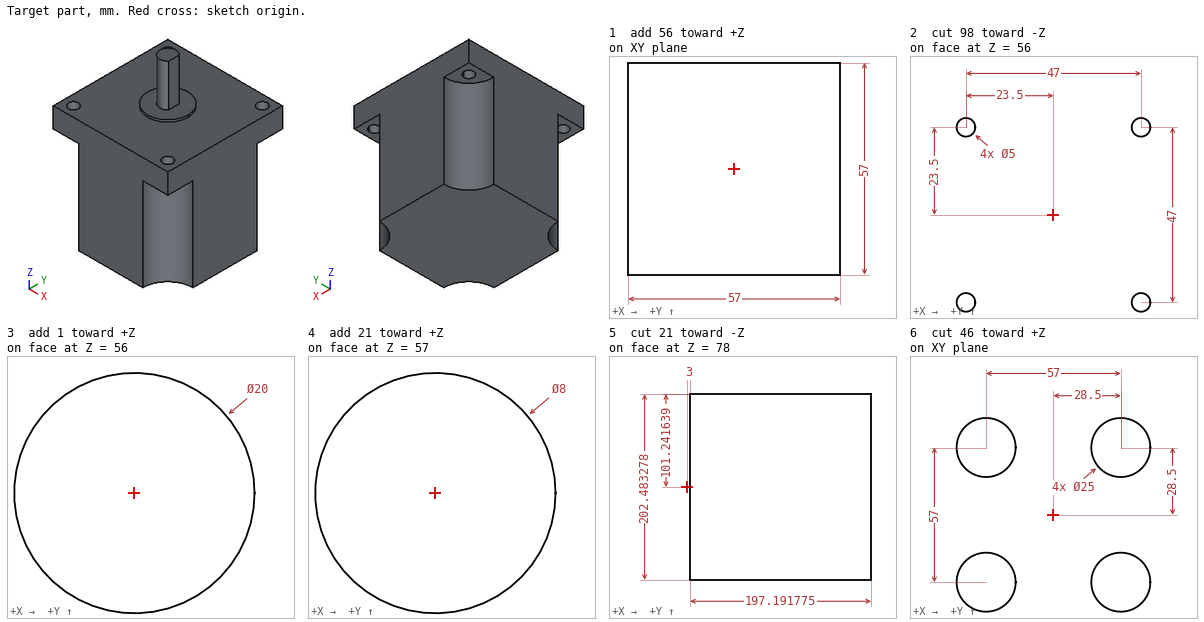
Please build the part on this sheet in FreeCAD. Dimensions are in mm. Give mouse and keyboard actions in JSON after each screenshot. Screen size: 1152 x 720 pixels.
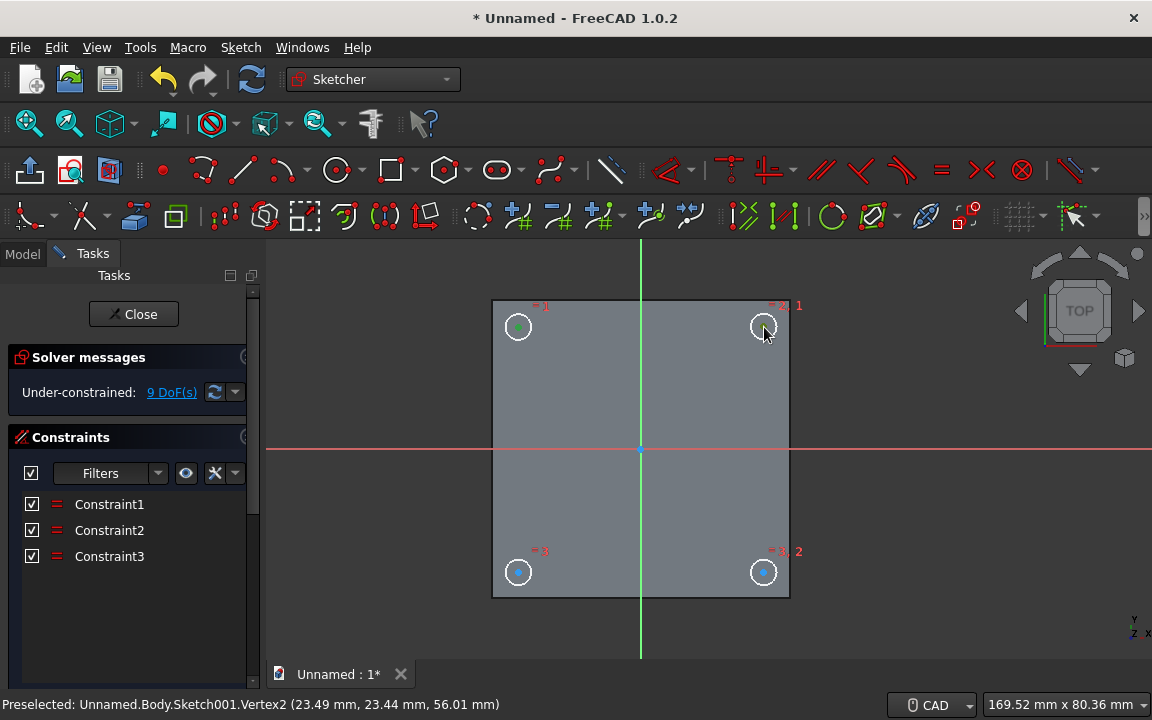
{"action": "key", "text": "h"}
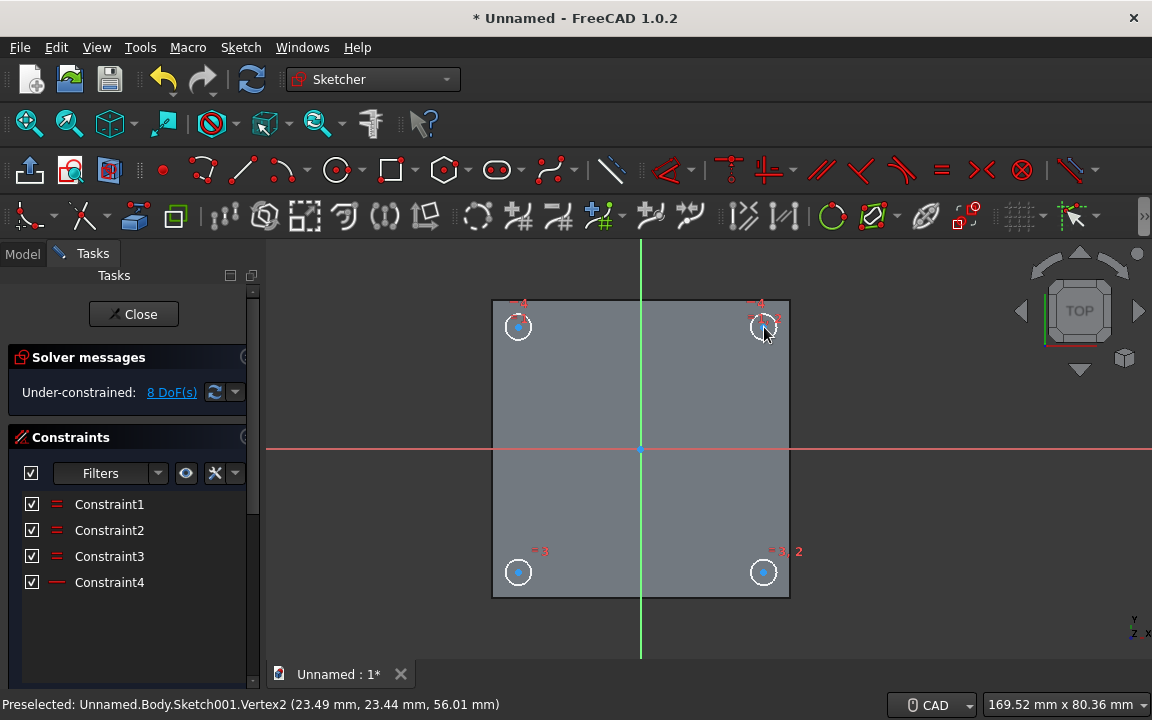
{"action": "left_click", "coordinate": [764, 327]}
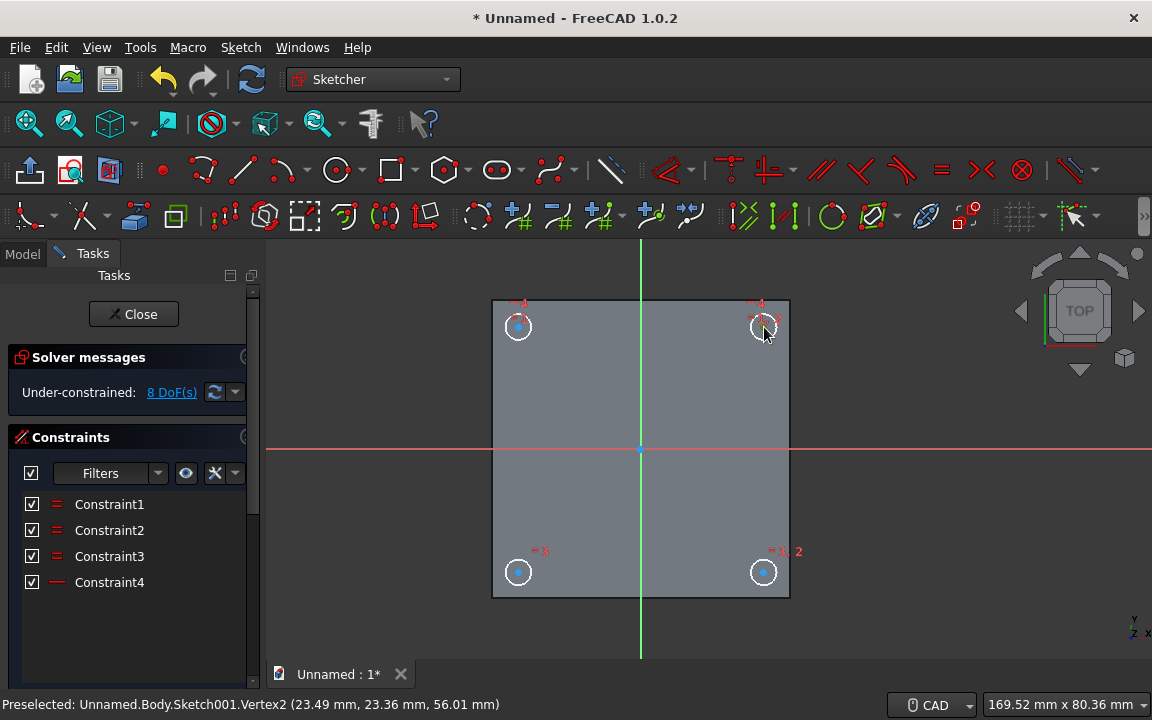
{"action": "left_click", "coordinate": [764, 572]}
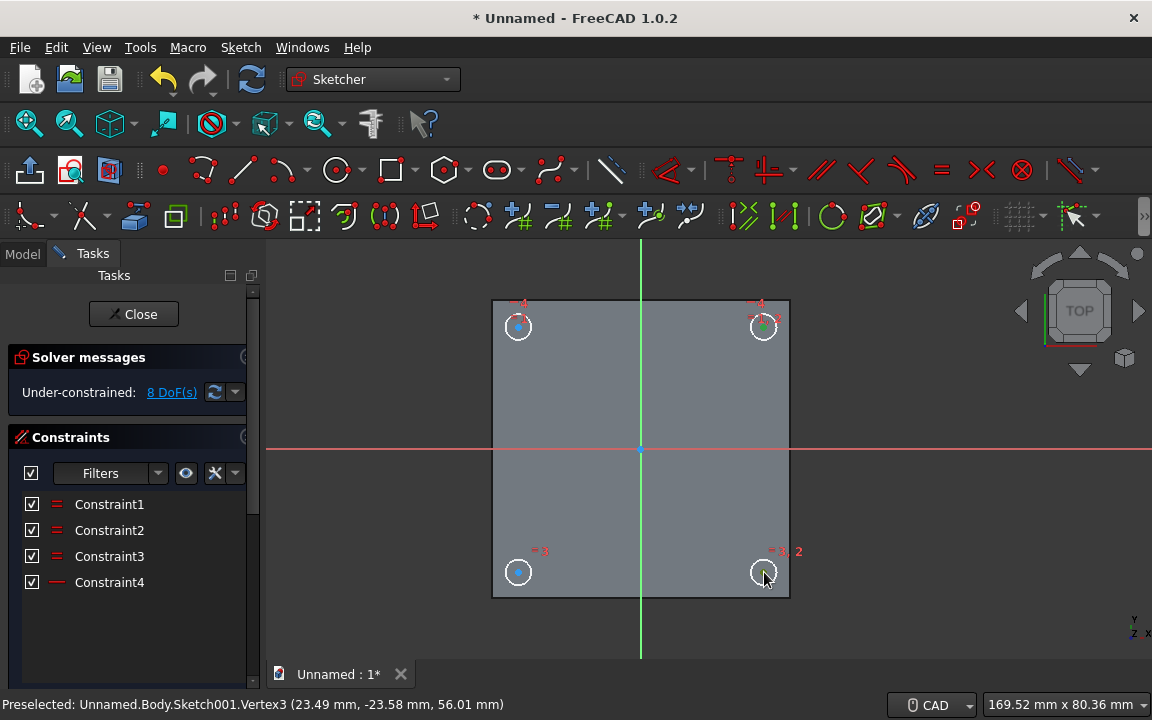
{"action": "key", "text": "v"}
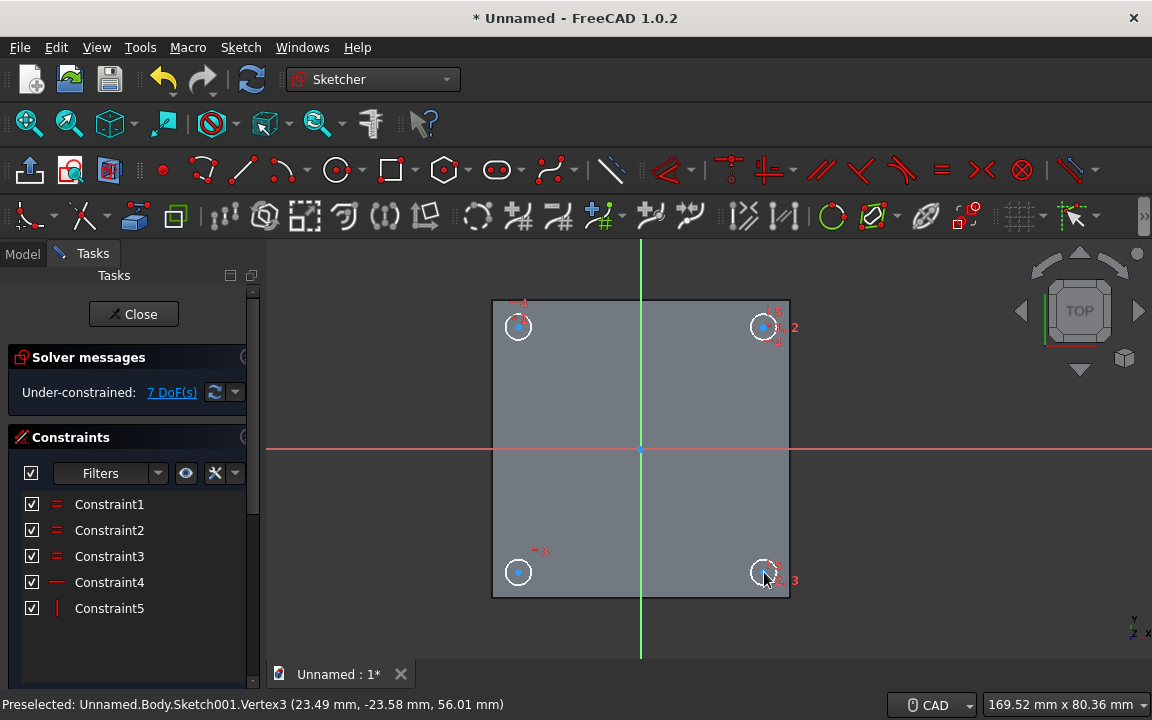
{"action": "left_click", "coordinate": [518, 327]}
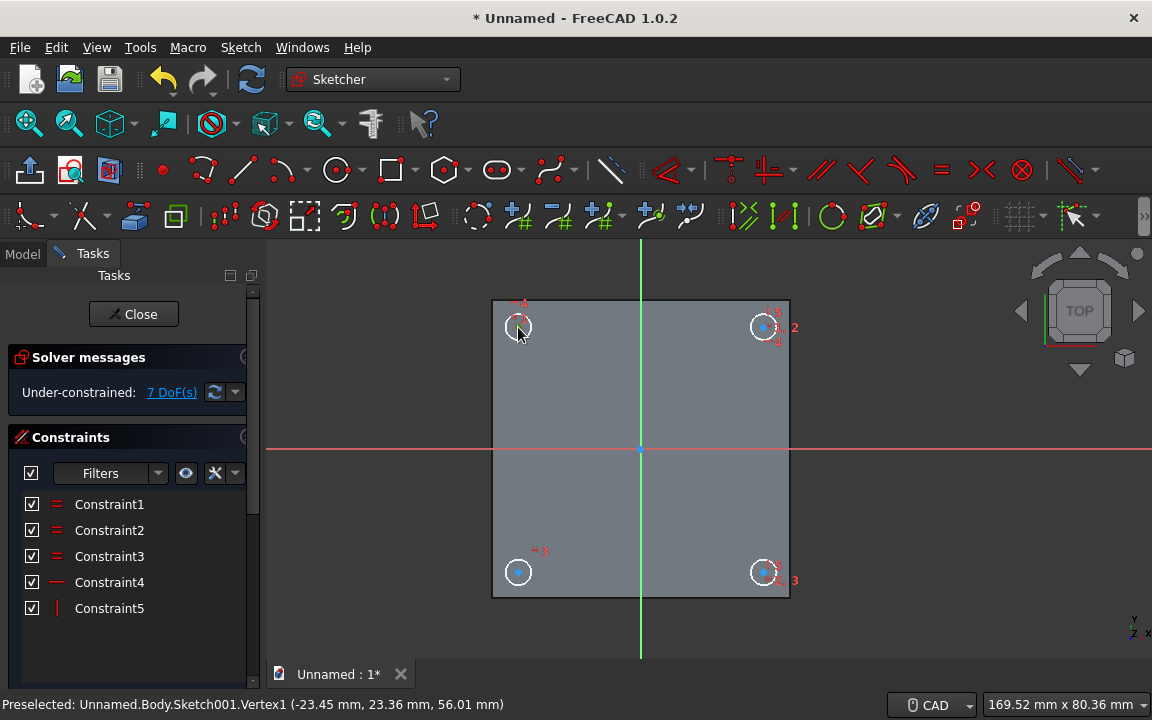
{"action": "left_click", "coordinate": [518, 572]}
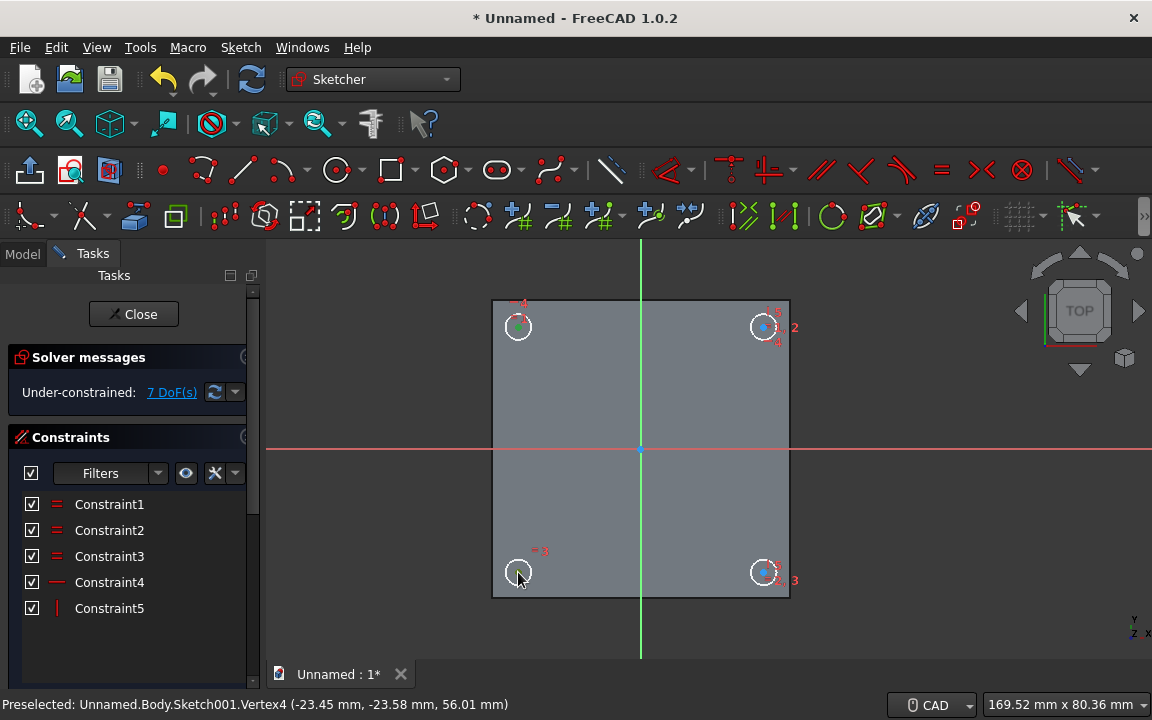
{"action": "left_click", "coordinate": [796, 170]}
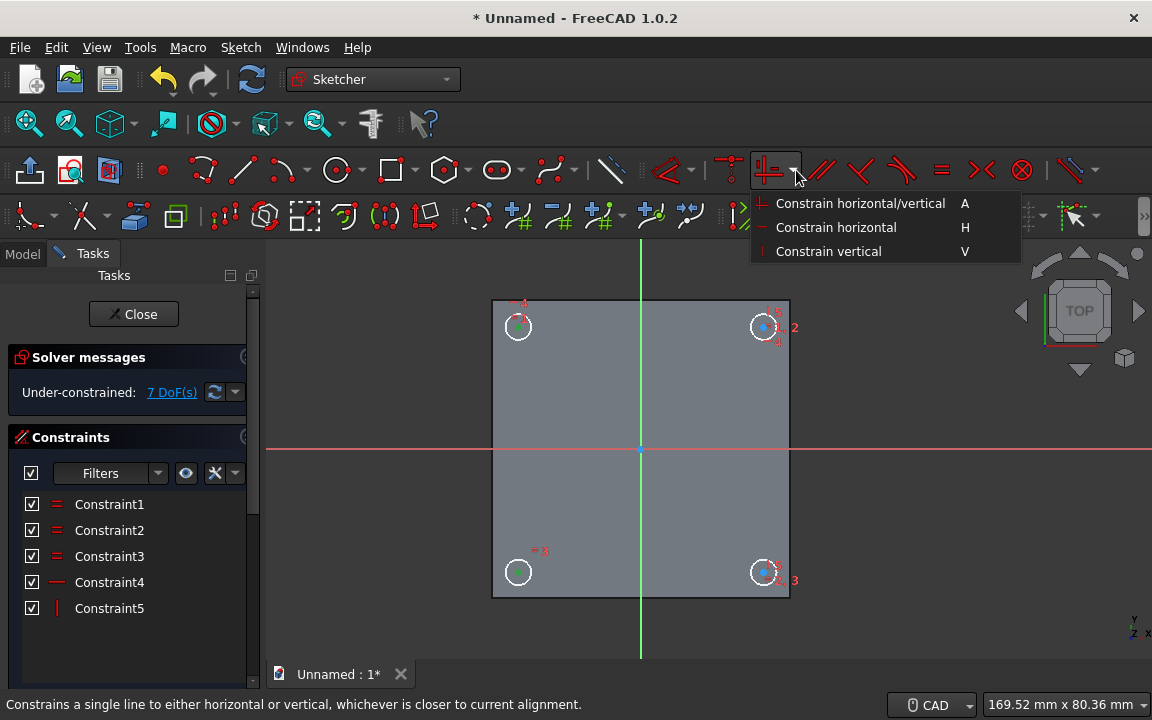
{"action": "left_click", "coordinate": [886, 251]}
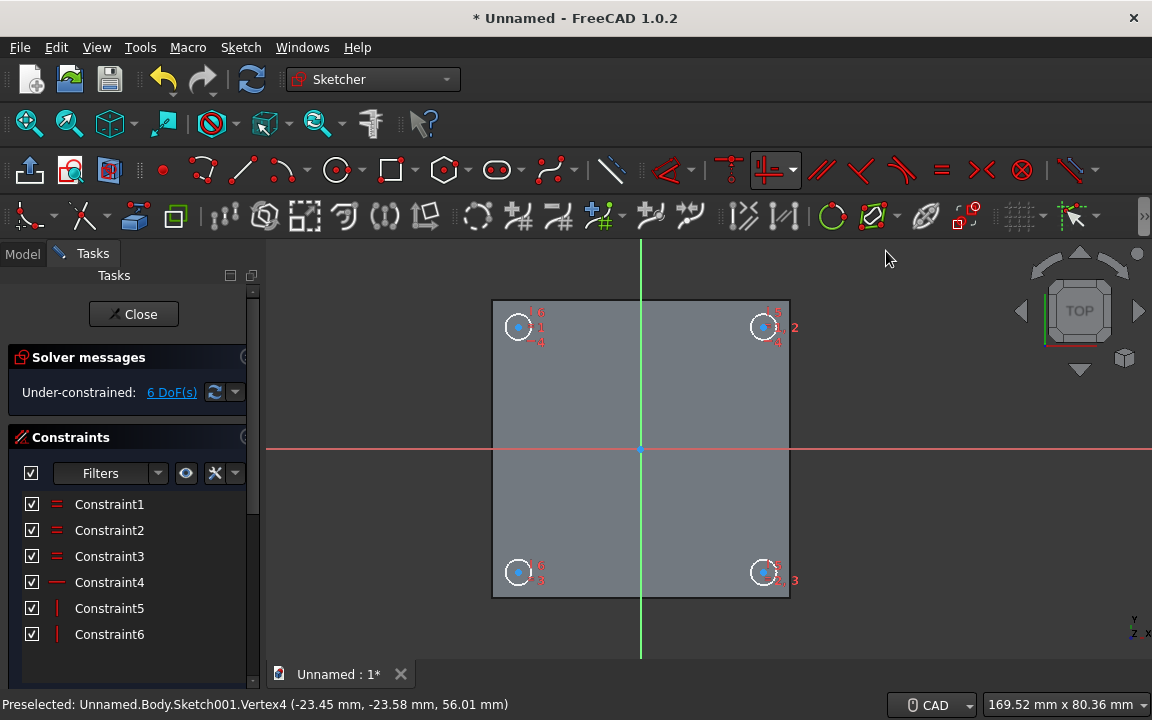
{"action": "left_click", "coordinate": [762, 574]}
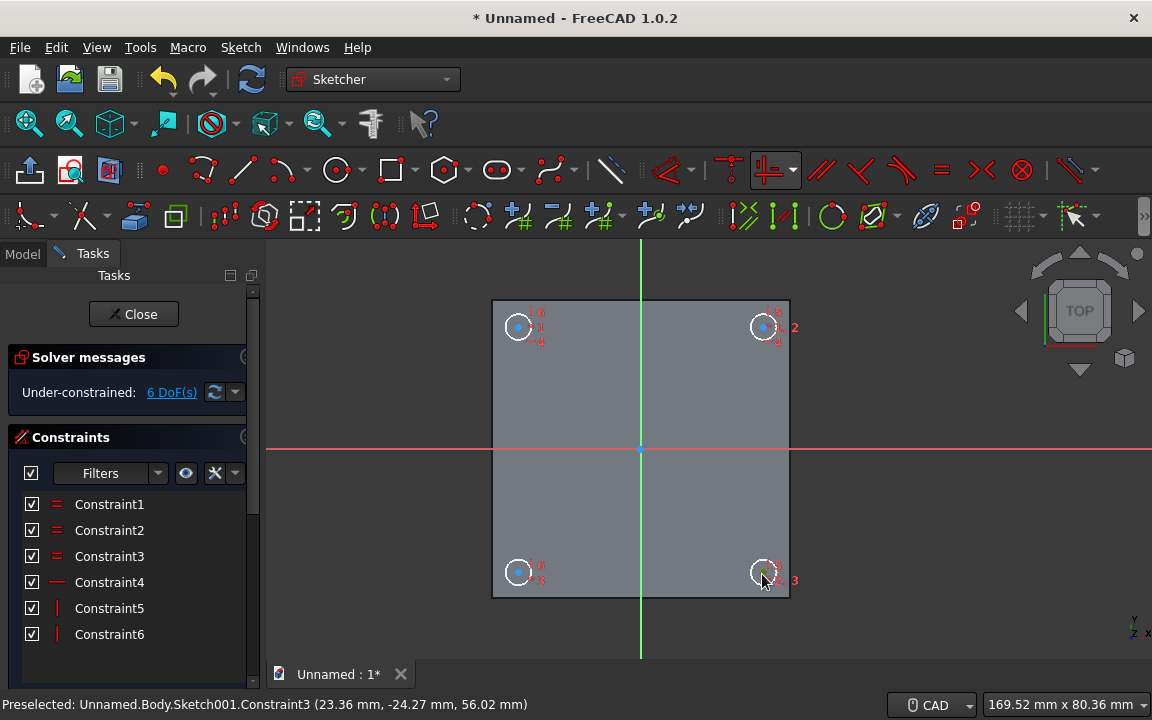
{"action": "left_click", "coordinate": [518, 572]}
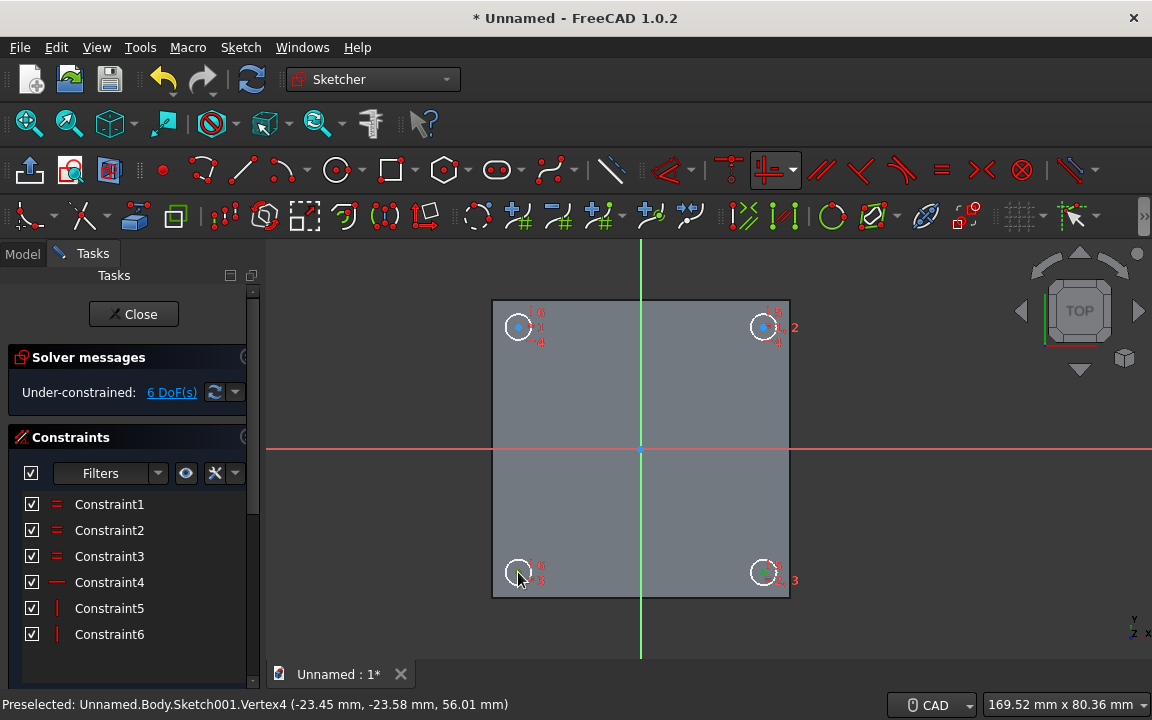
{"action": "left_click", "coordinate": [796, 170]}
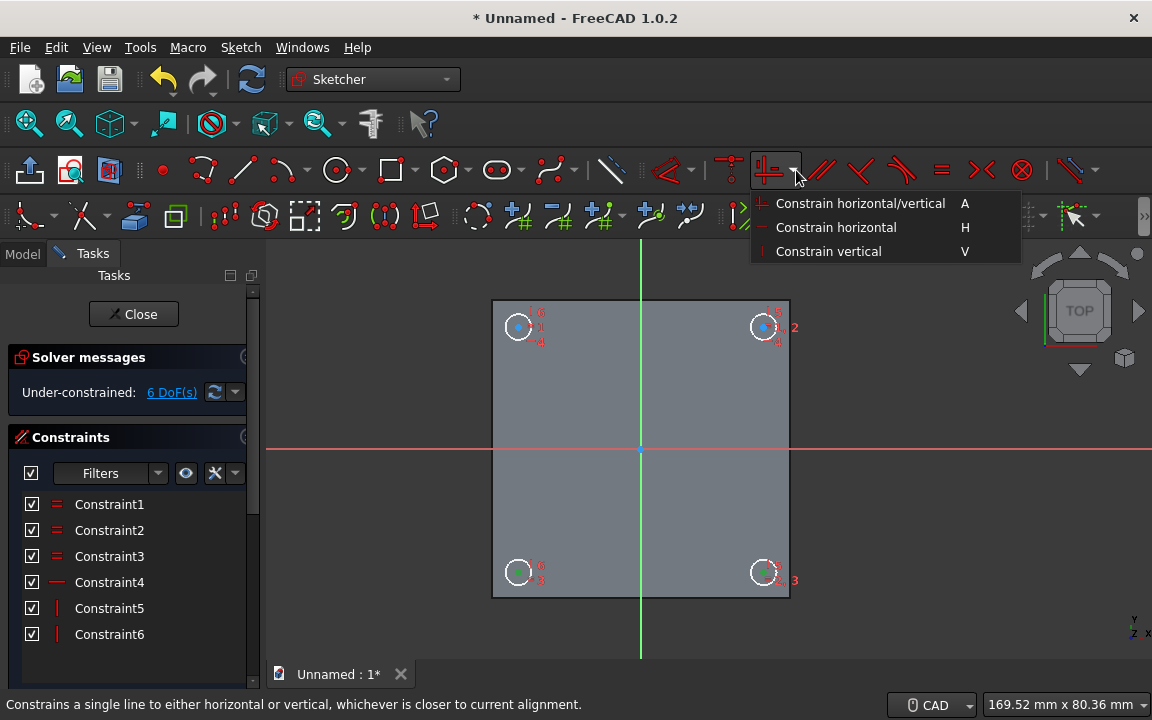
{"action": "left_click", "coordinate": [886, 227]}